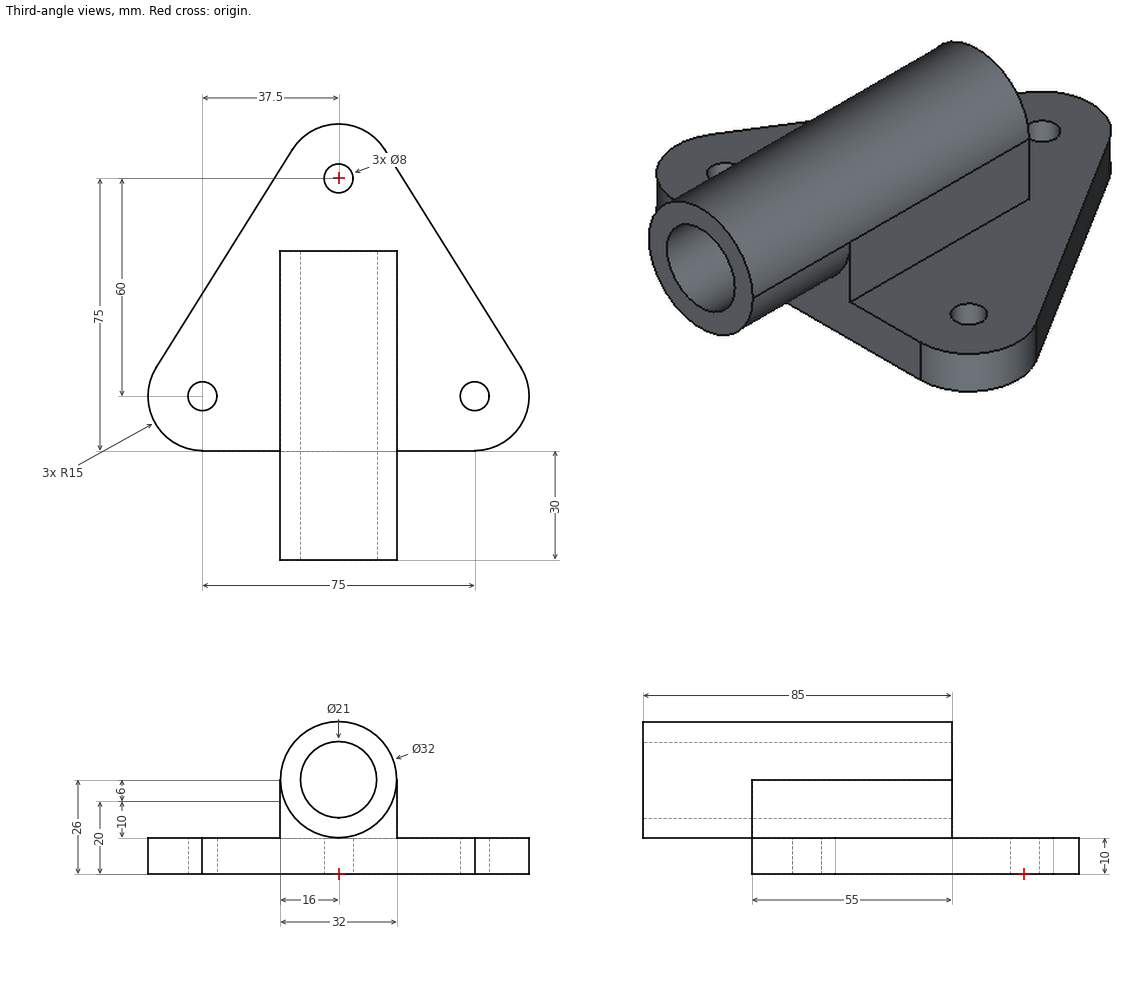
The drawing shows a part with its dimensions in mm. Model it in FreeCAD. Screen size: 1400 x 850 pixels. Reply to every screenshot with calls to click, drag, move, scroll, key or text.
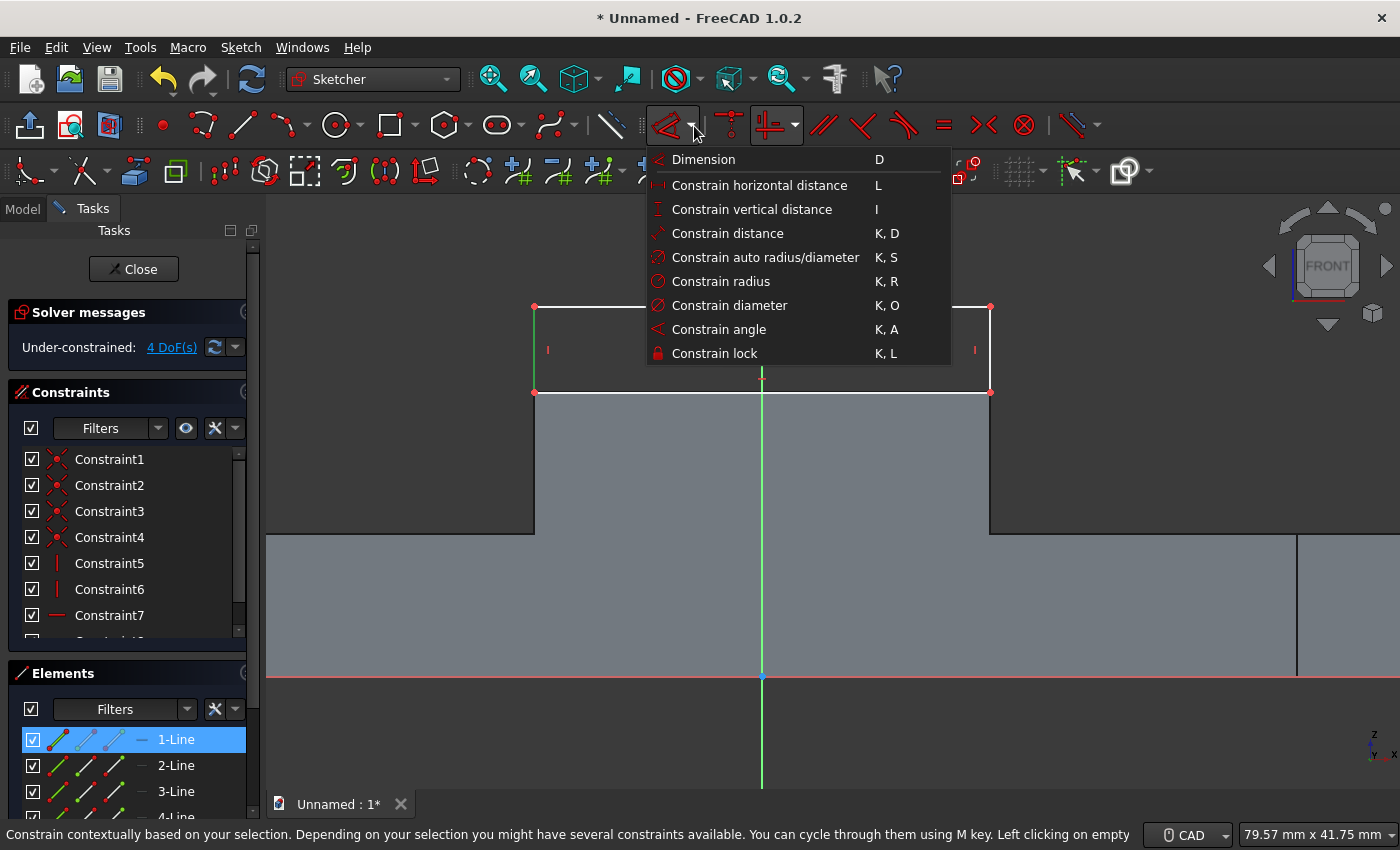
click(799, 209)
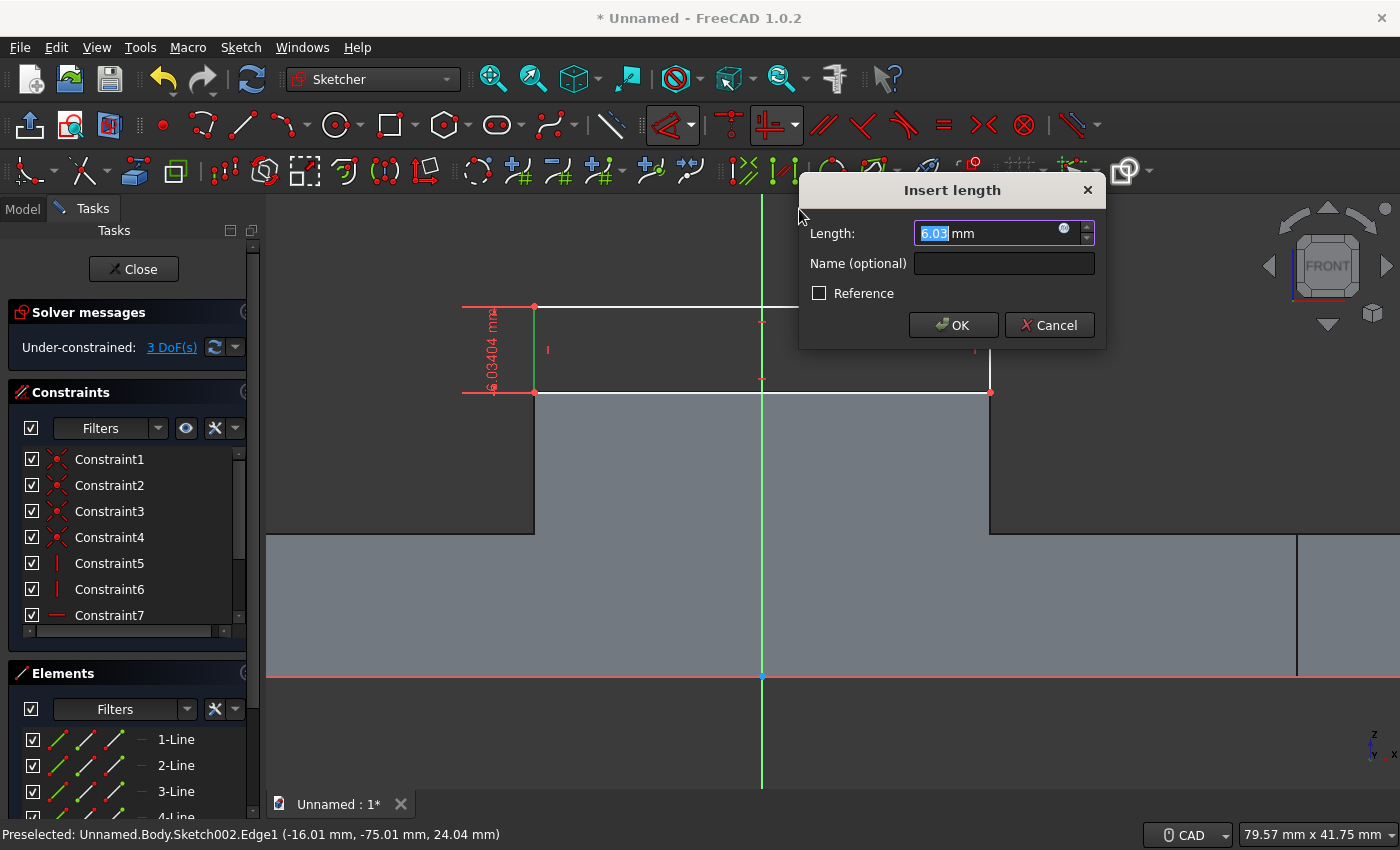
text(6)
key(Return)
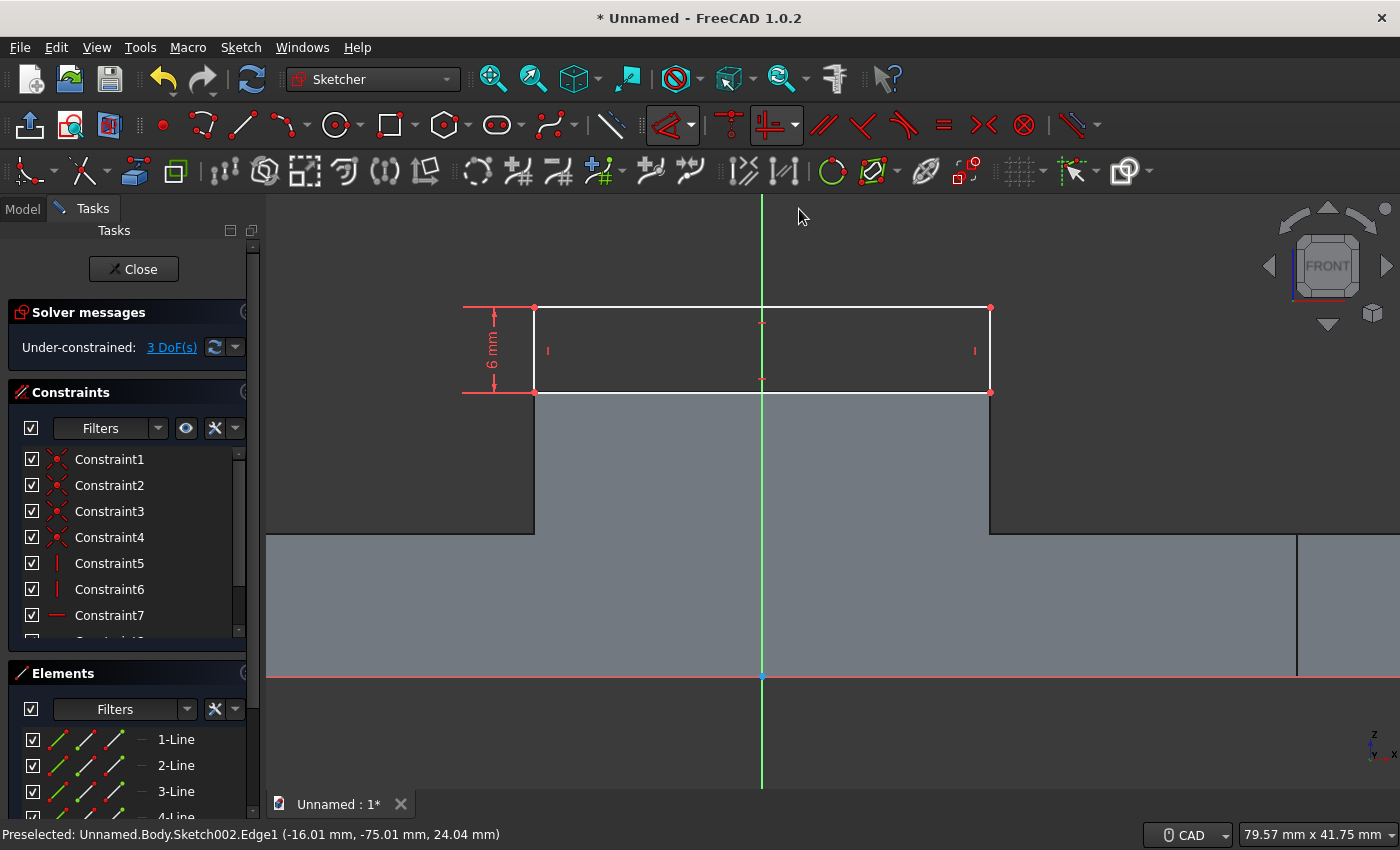
click(671, 393)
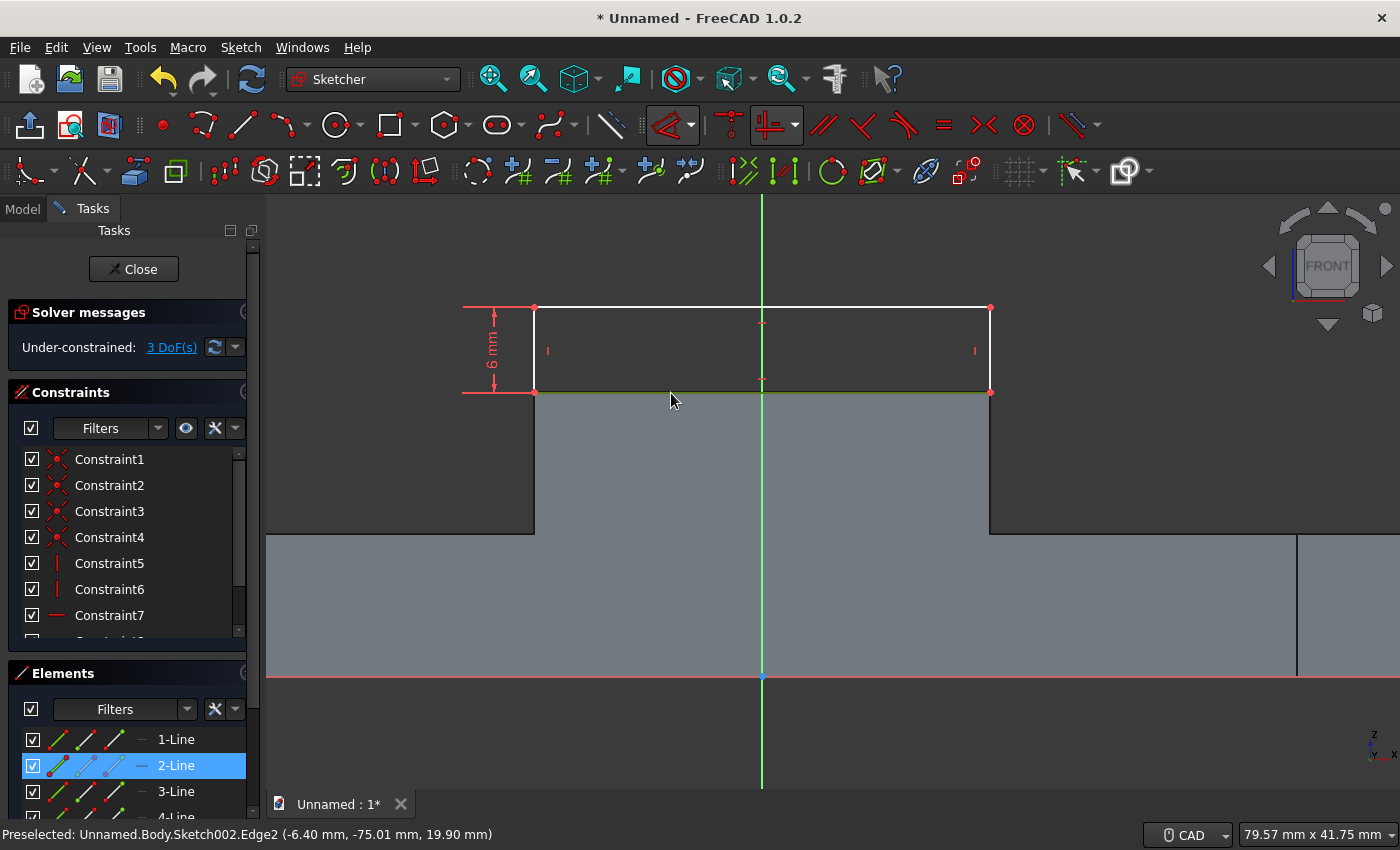
key(l)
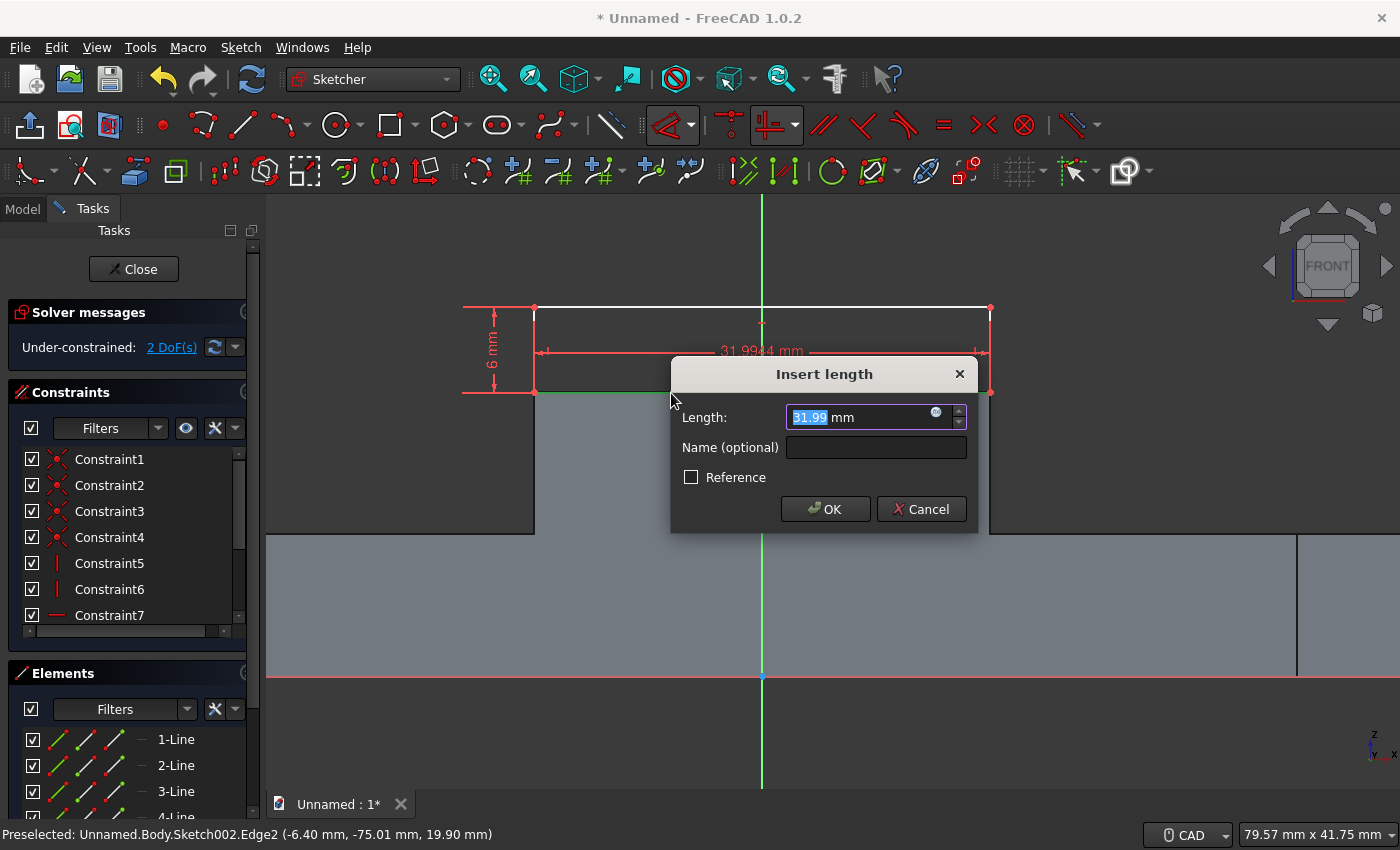
text(32)
key(Return)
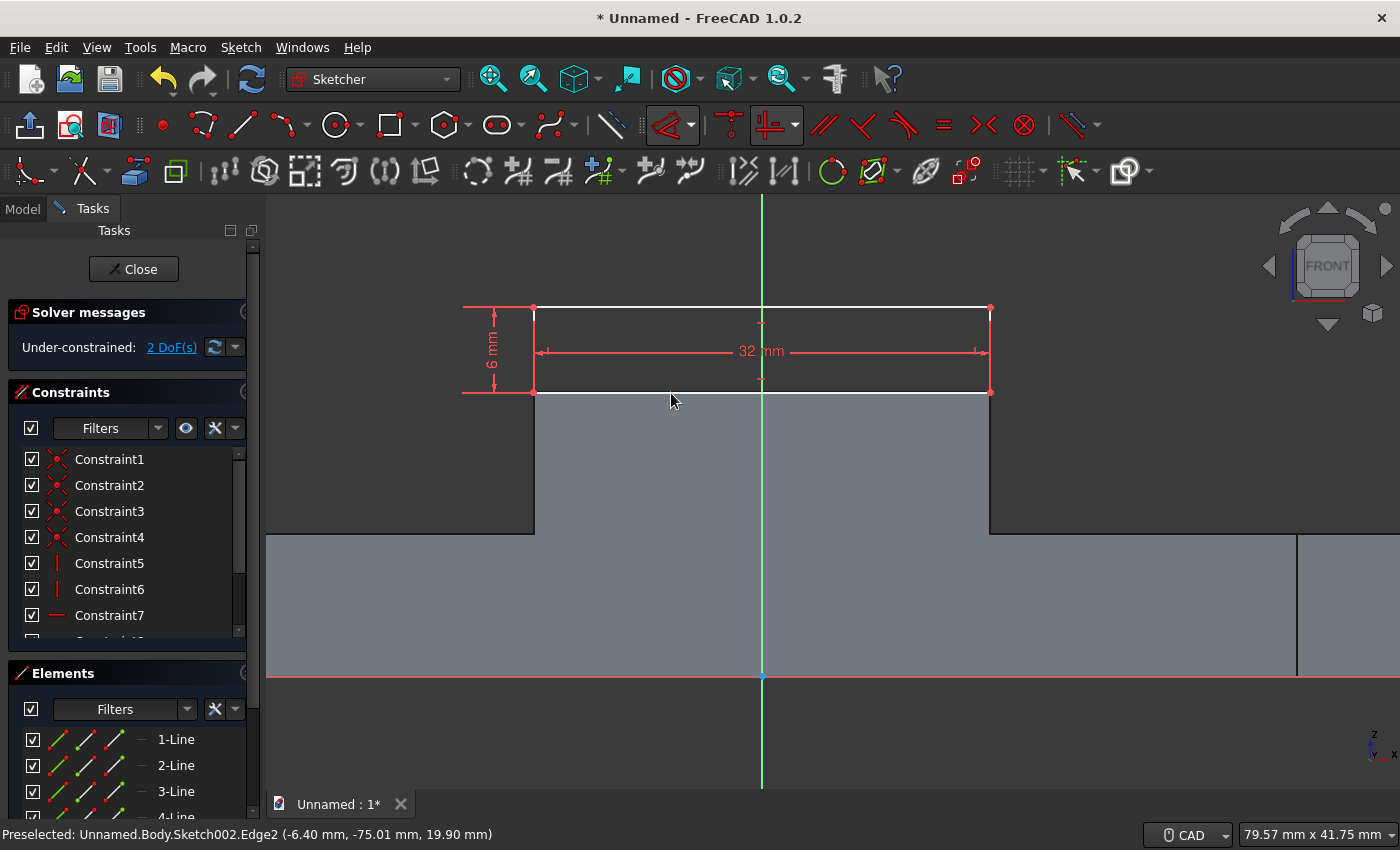
click(534, 307)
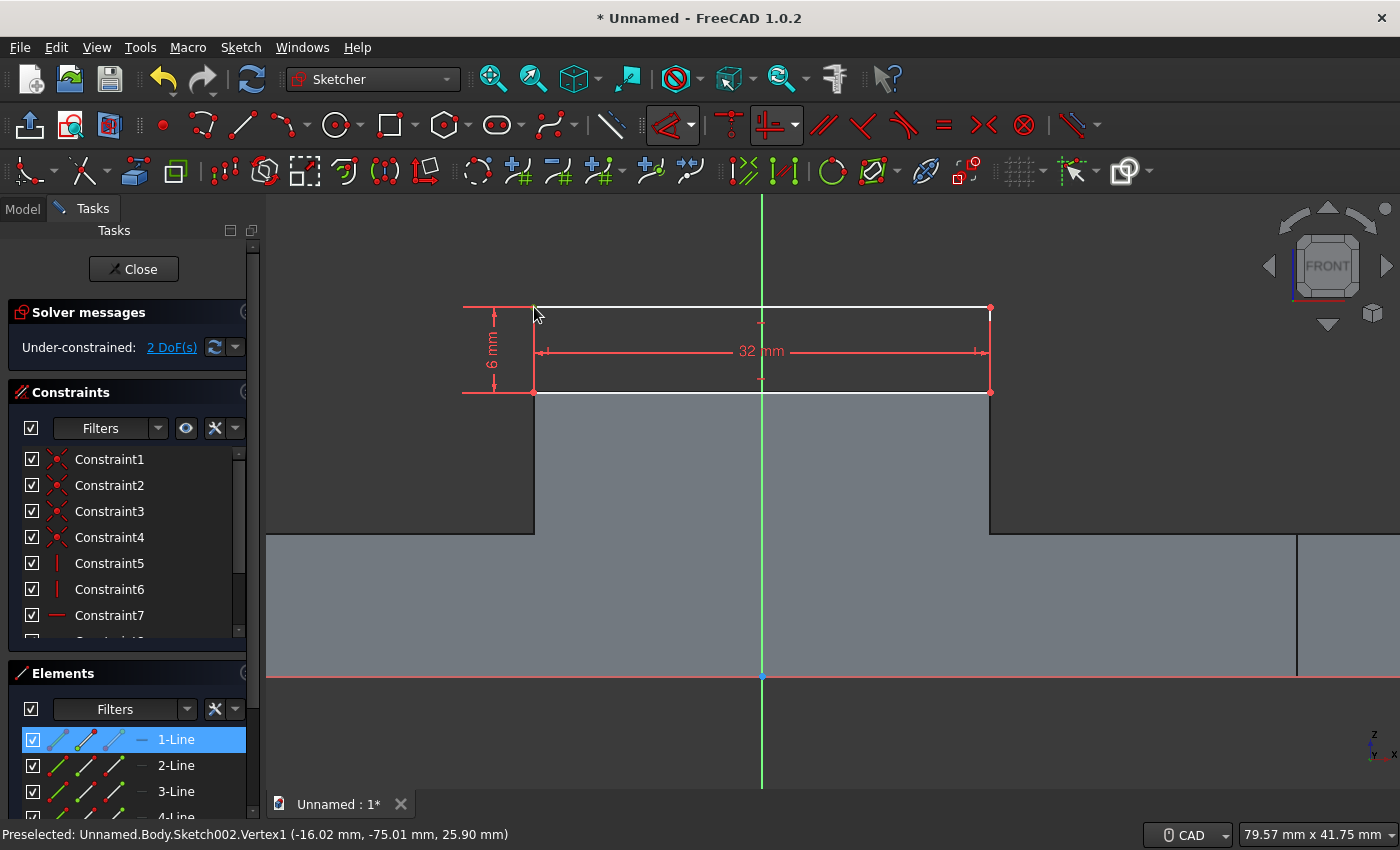
click(694, 126)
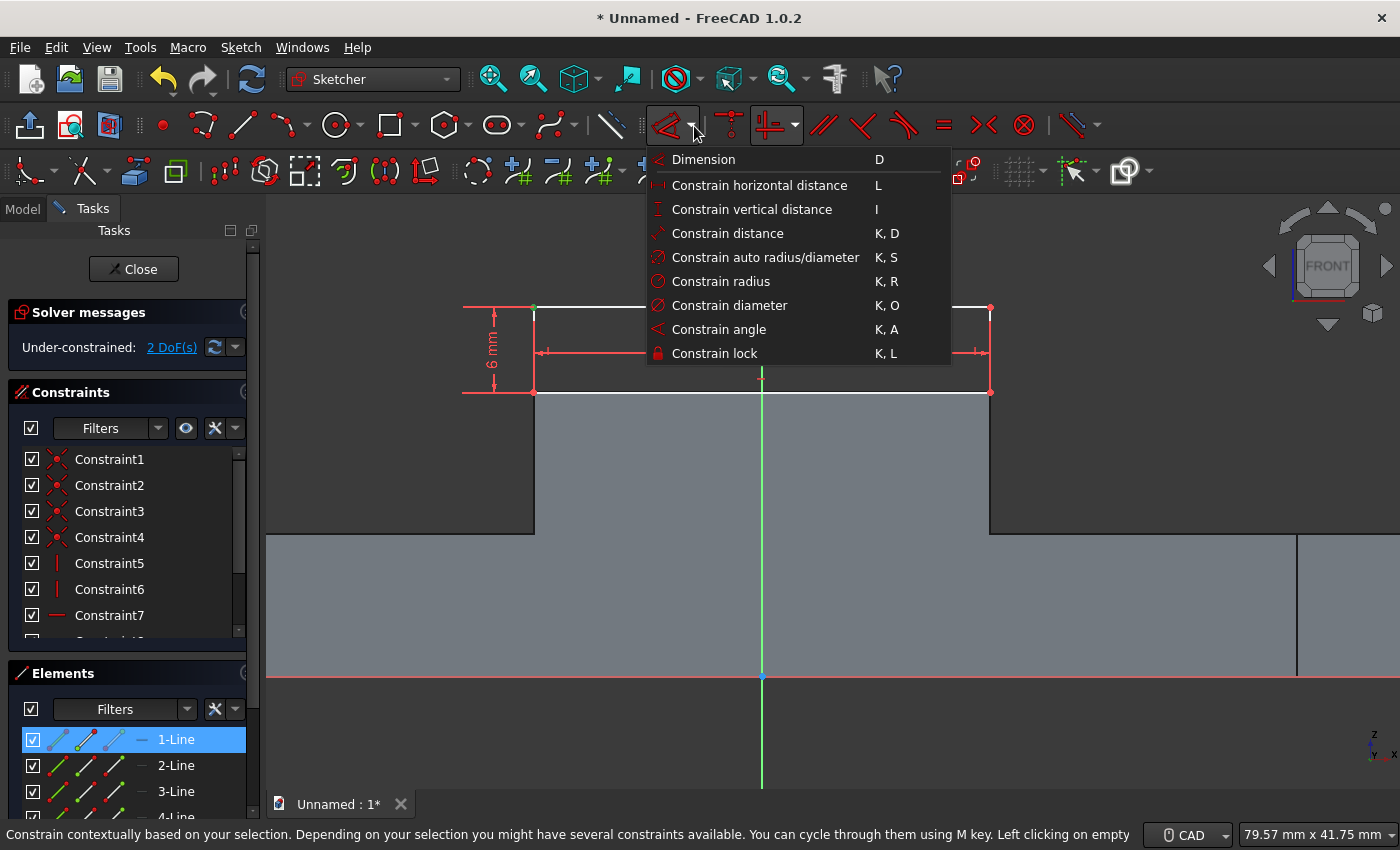
click(799, 185)